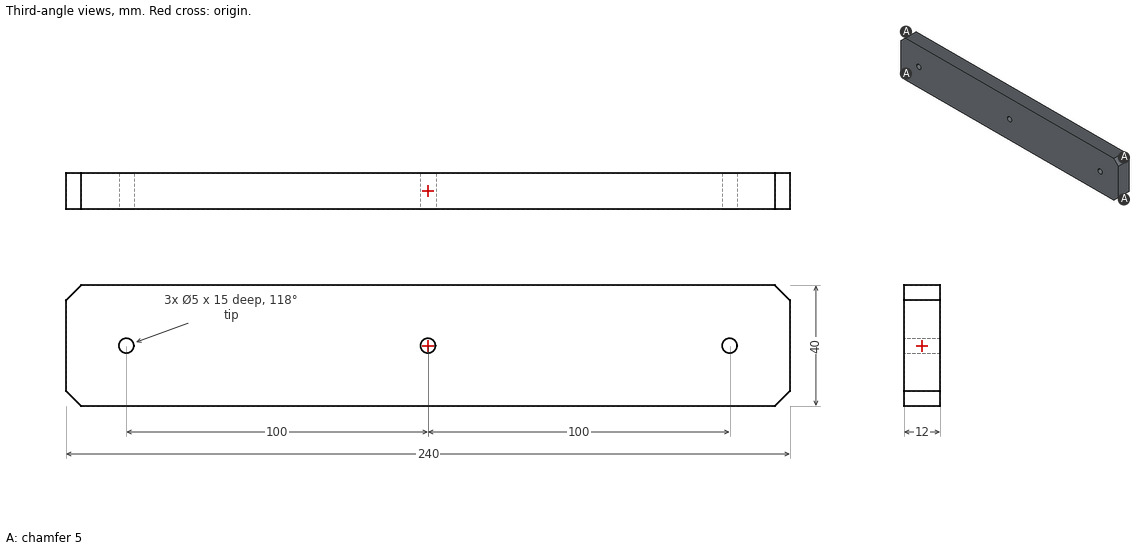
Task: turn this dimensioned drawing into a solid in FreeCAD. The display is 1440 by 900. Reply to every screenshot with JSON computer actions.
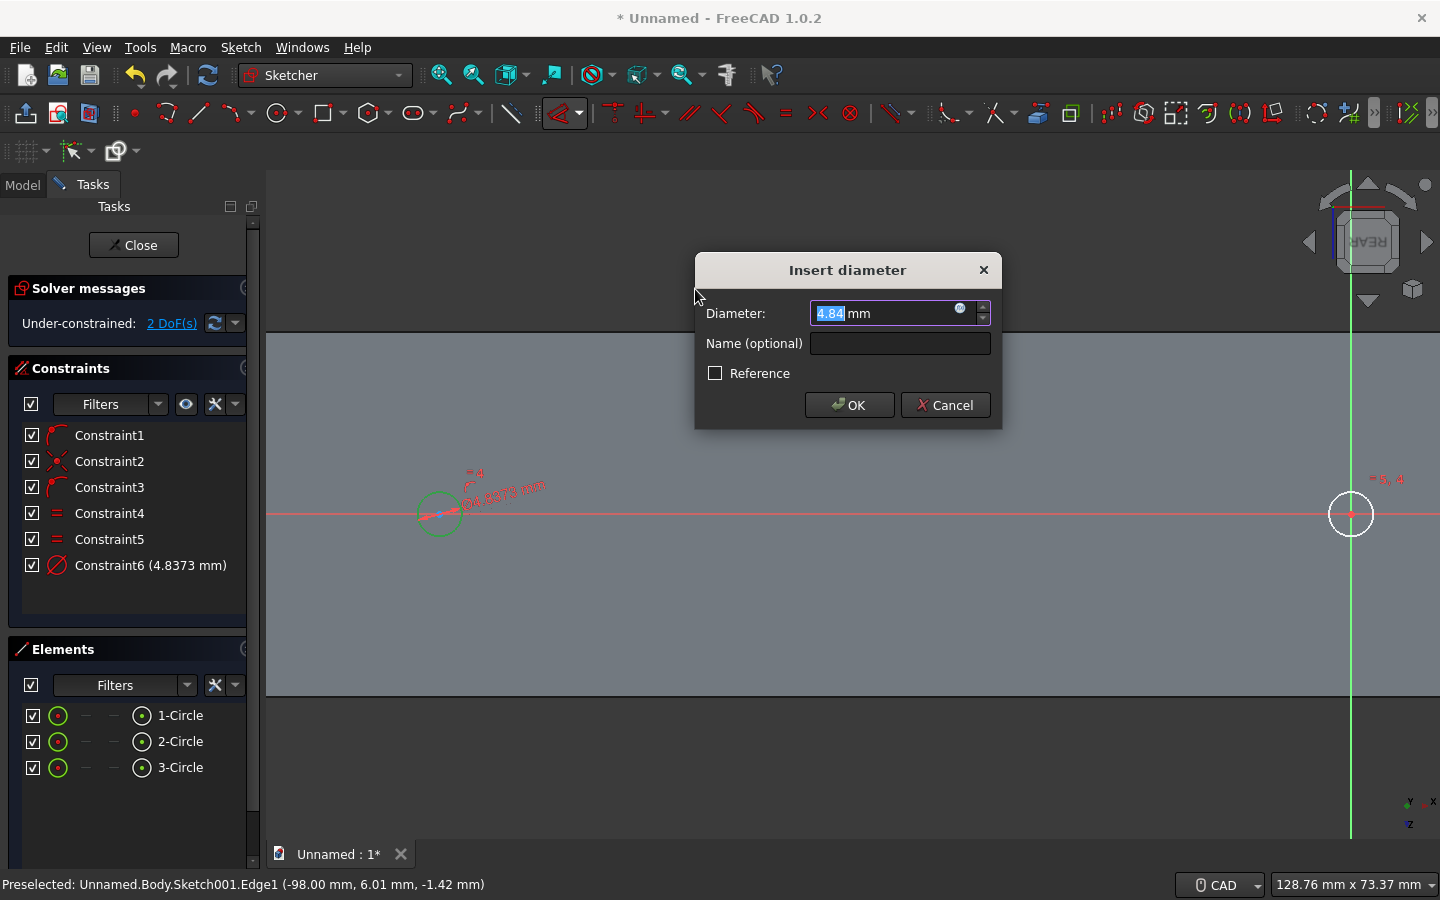
{"action": "type", "text": "5"}
{"action": "key", "text": "Return"}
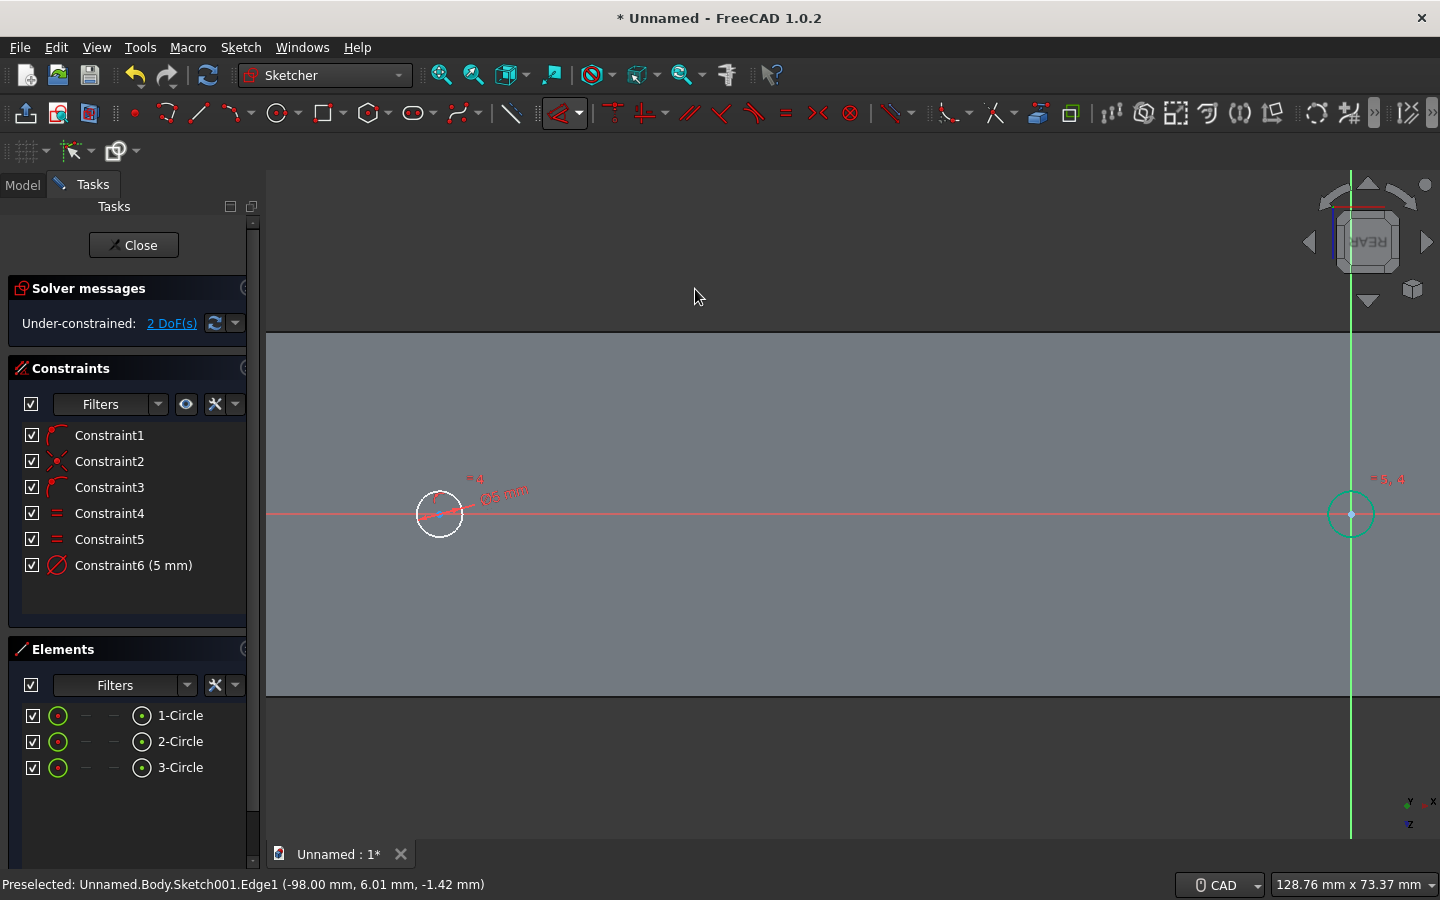
{"action": "left_click", "coordinate": [440, 514]}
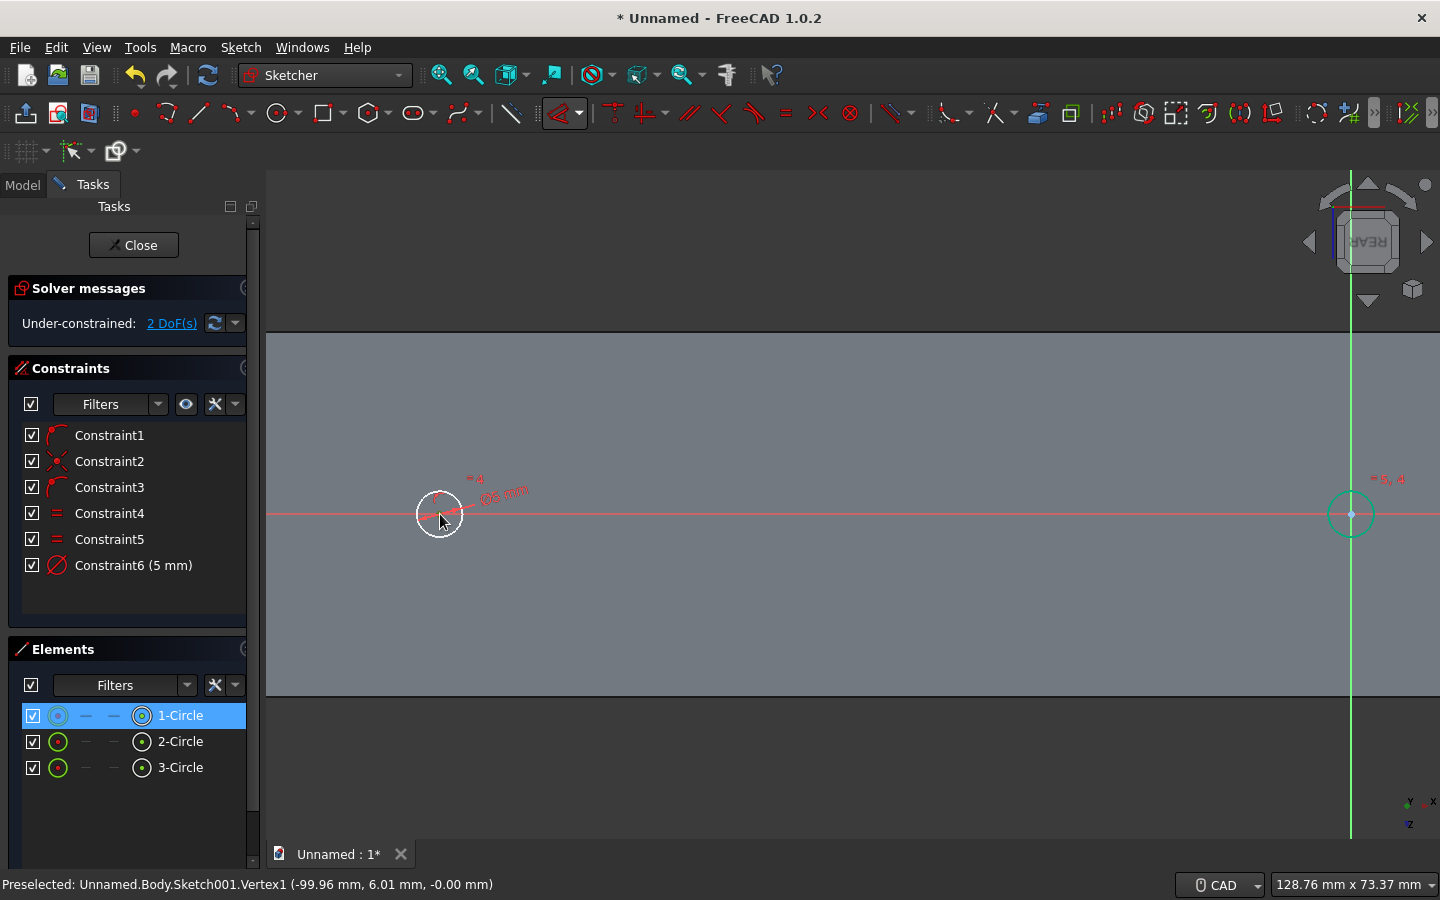
{"action": "key", "text": "l"}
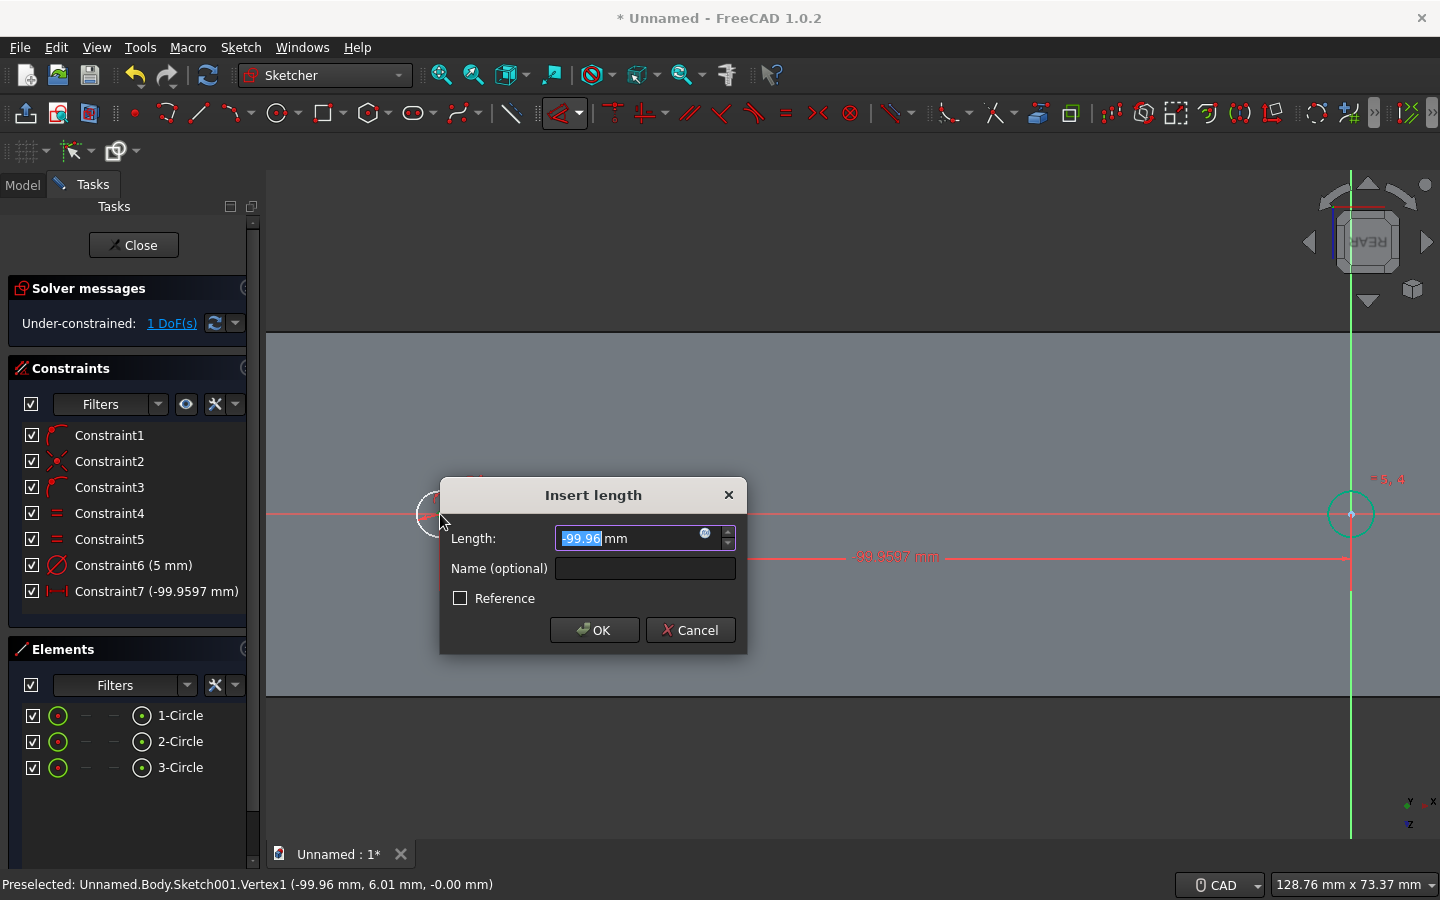
{"action": "type", "text": "-100"}
{"action": "key", "text": "Return"}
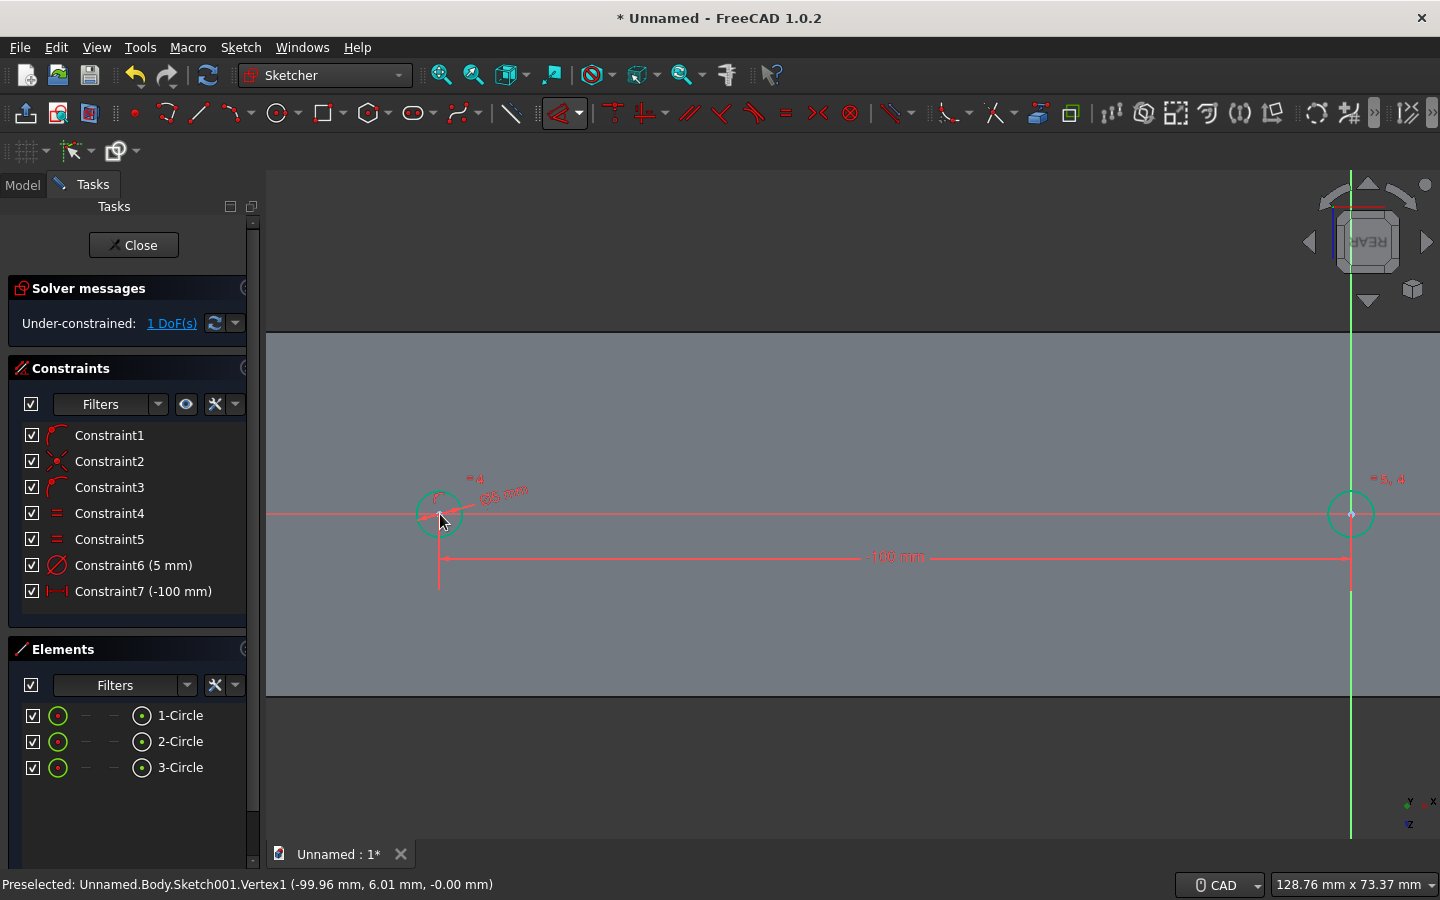
{"action": "scroll", "coordinate": [455, 499], "scroll_direction": "down", "scroll_amount": 5}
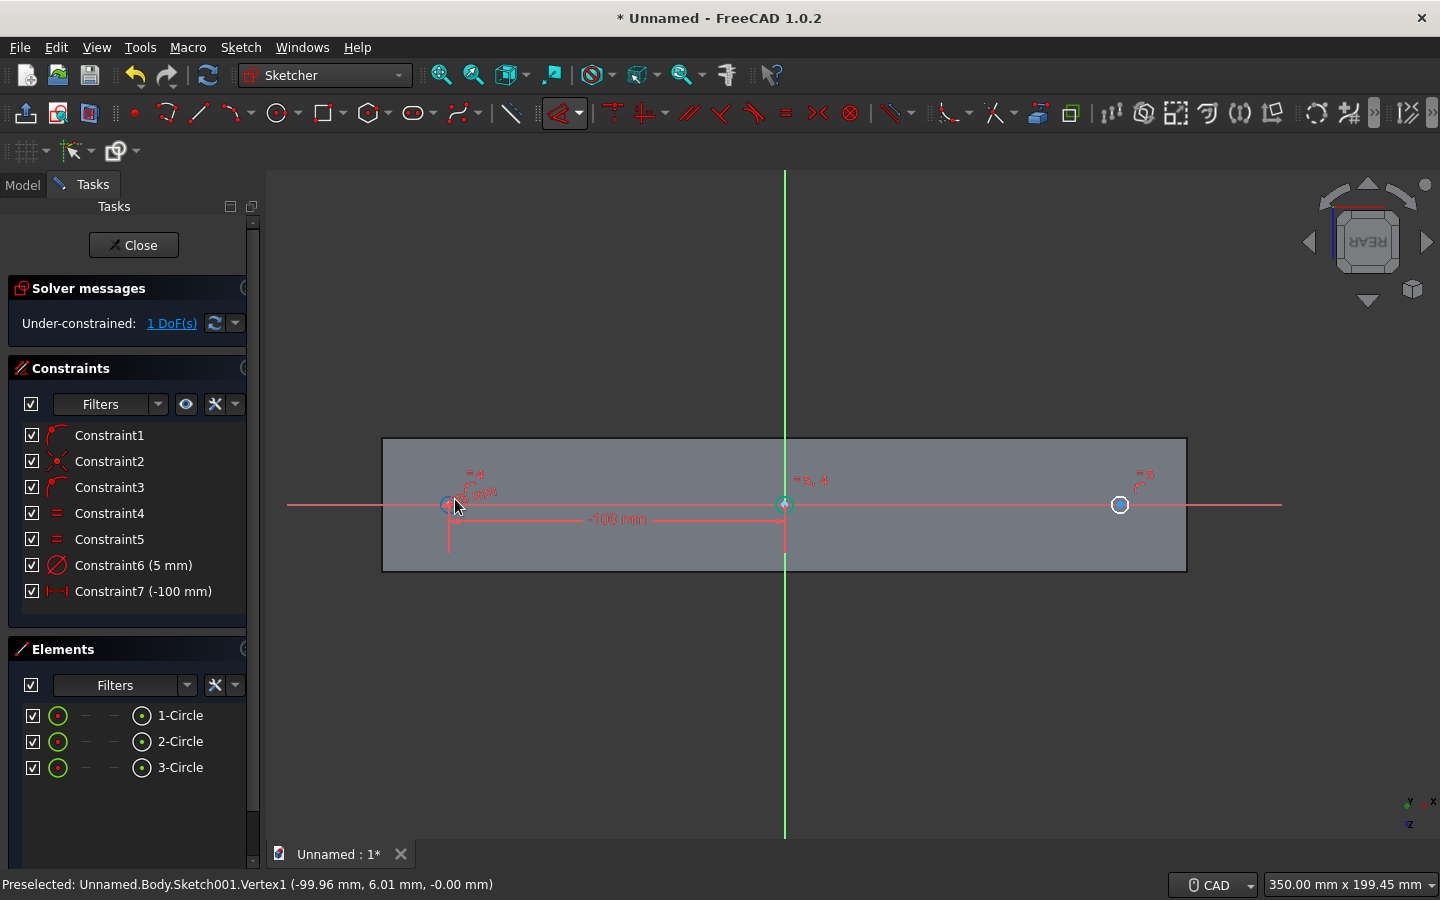
{"action": "left_click", "coordinate": [1120, 505]}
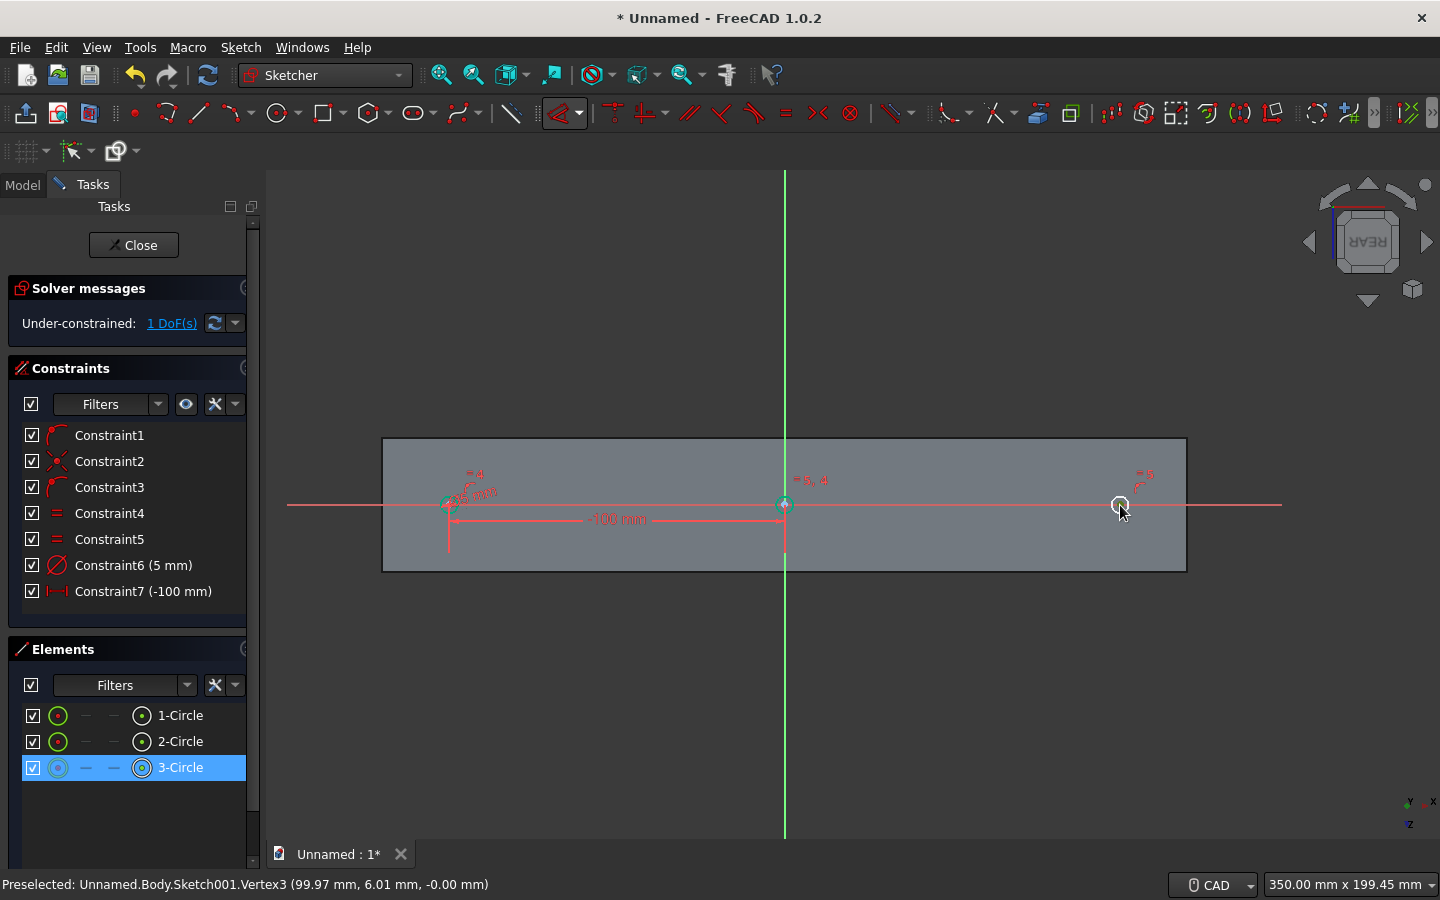
{"action": "key", "text": "l"}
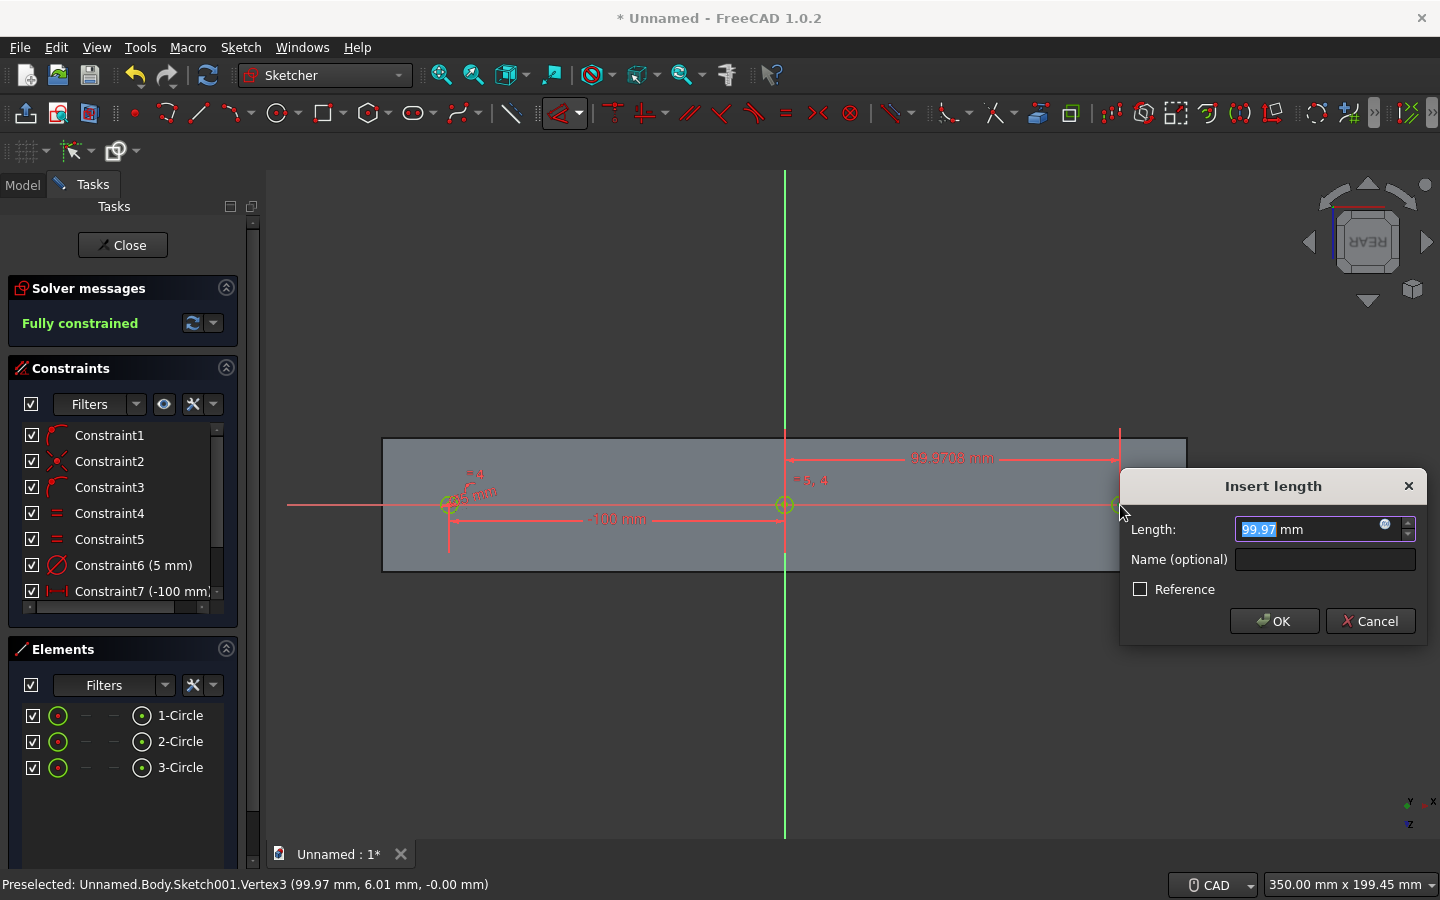
{"action": "type", "text": "100"}
{"action": "key", "text": "Return"}